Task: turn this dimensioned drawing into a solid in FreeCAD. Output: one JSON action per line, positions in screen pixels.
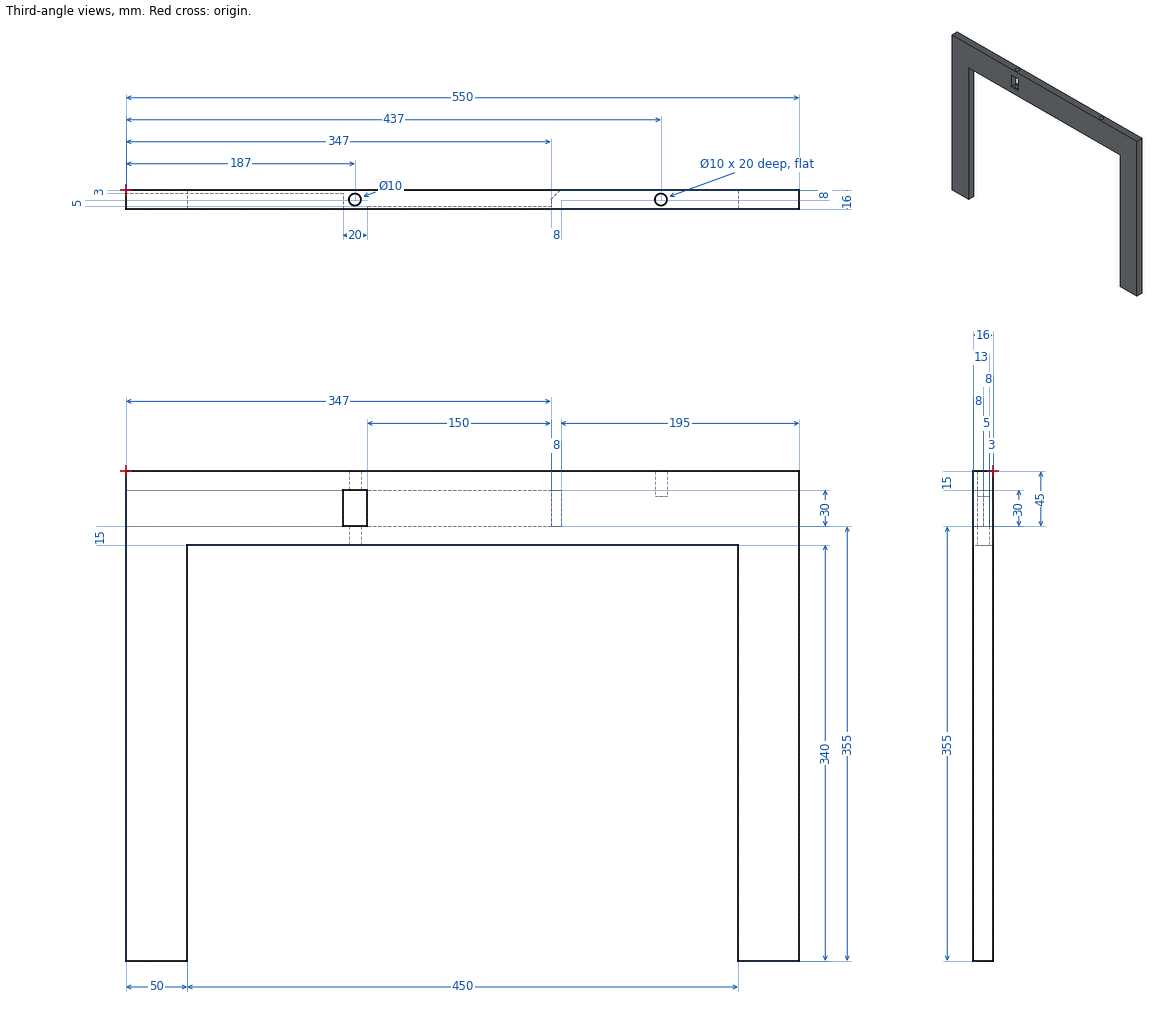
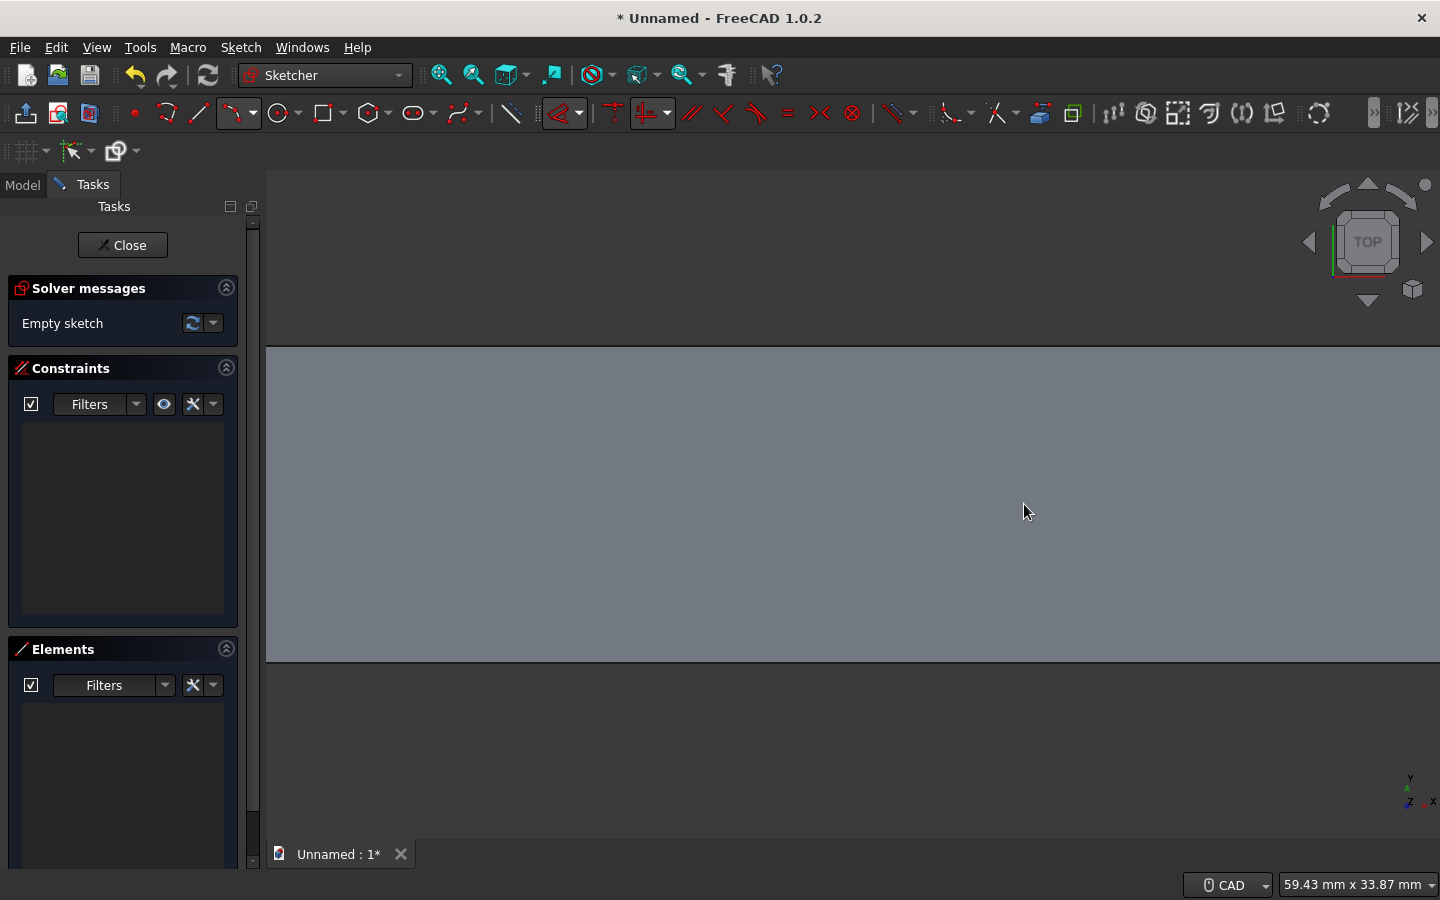
{"action": "scroll", "coordinate": [771, 504], "scroll_direction": "up", "scroll_amount": 4}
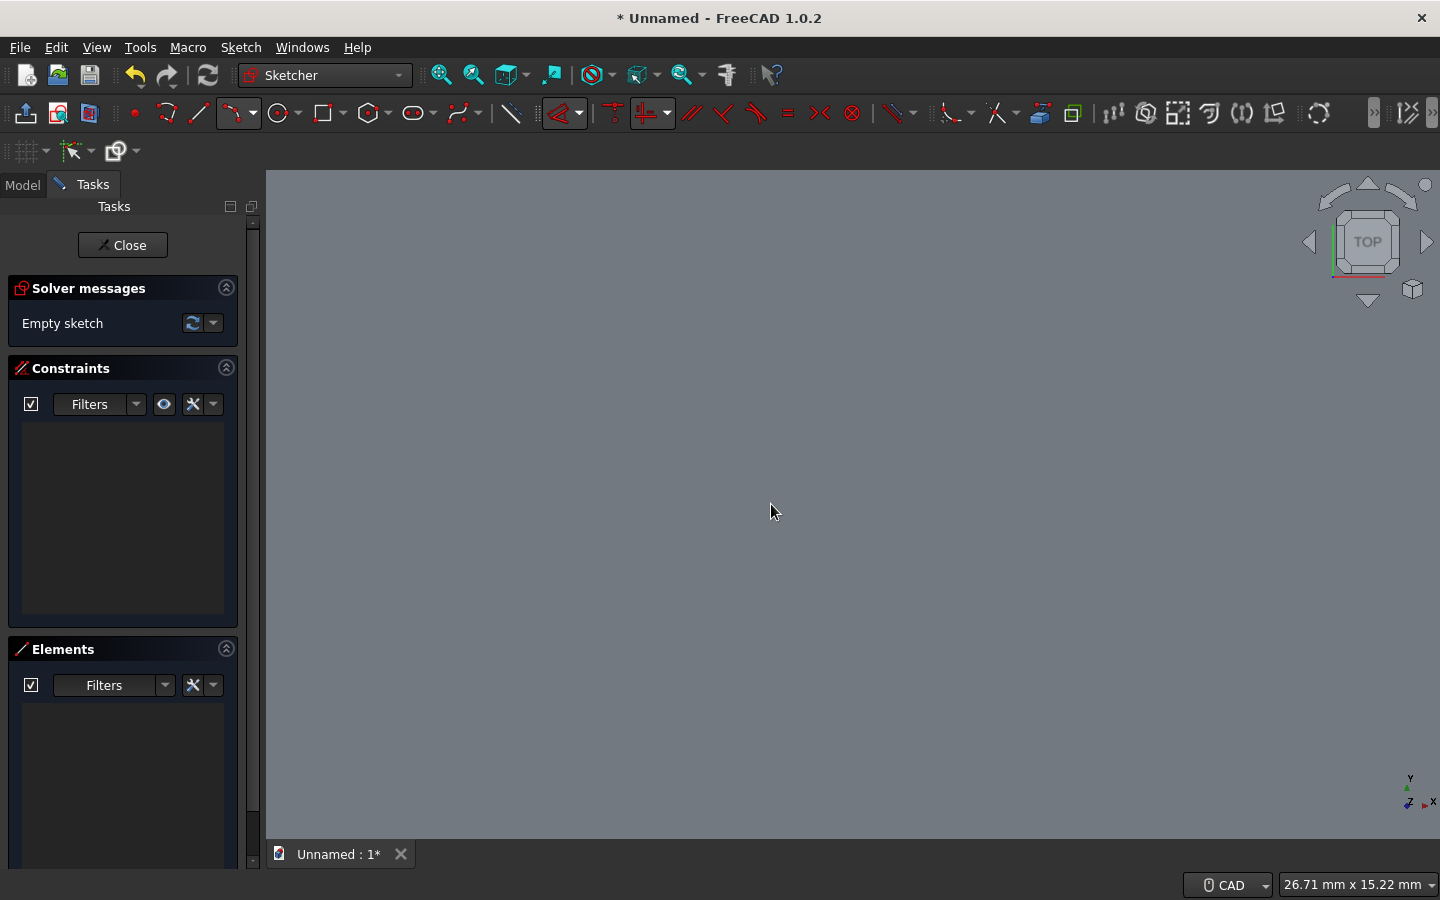
{"action": "left_click", "coordinate": [278, 114]}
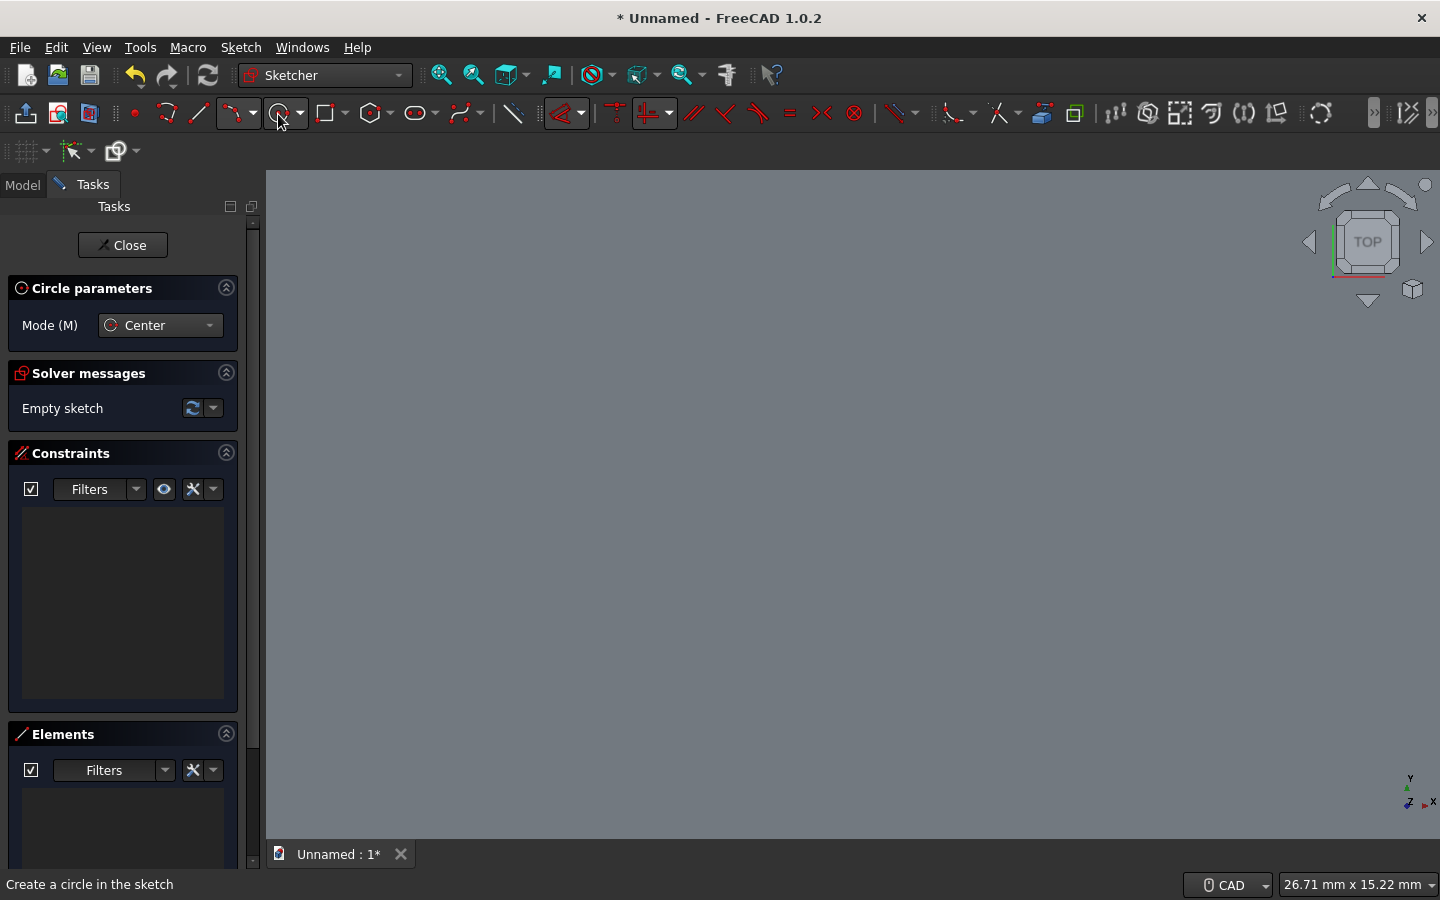
{"action": "left_click", "coordinate": [784, 504]}
{"action": "left_click", "coordinate": [939, 349]}
{"action": "key", "text": "Escape"}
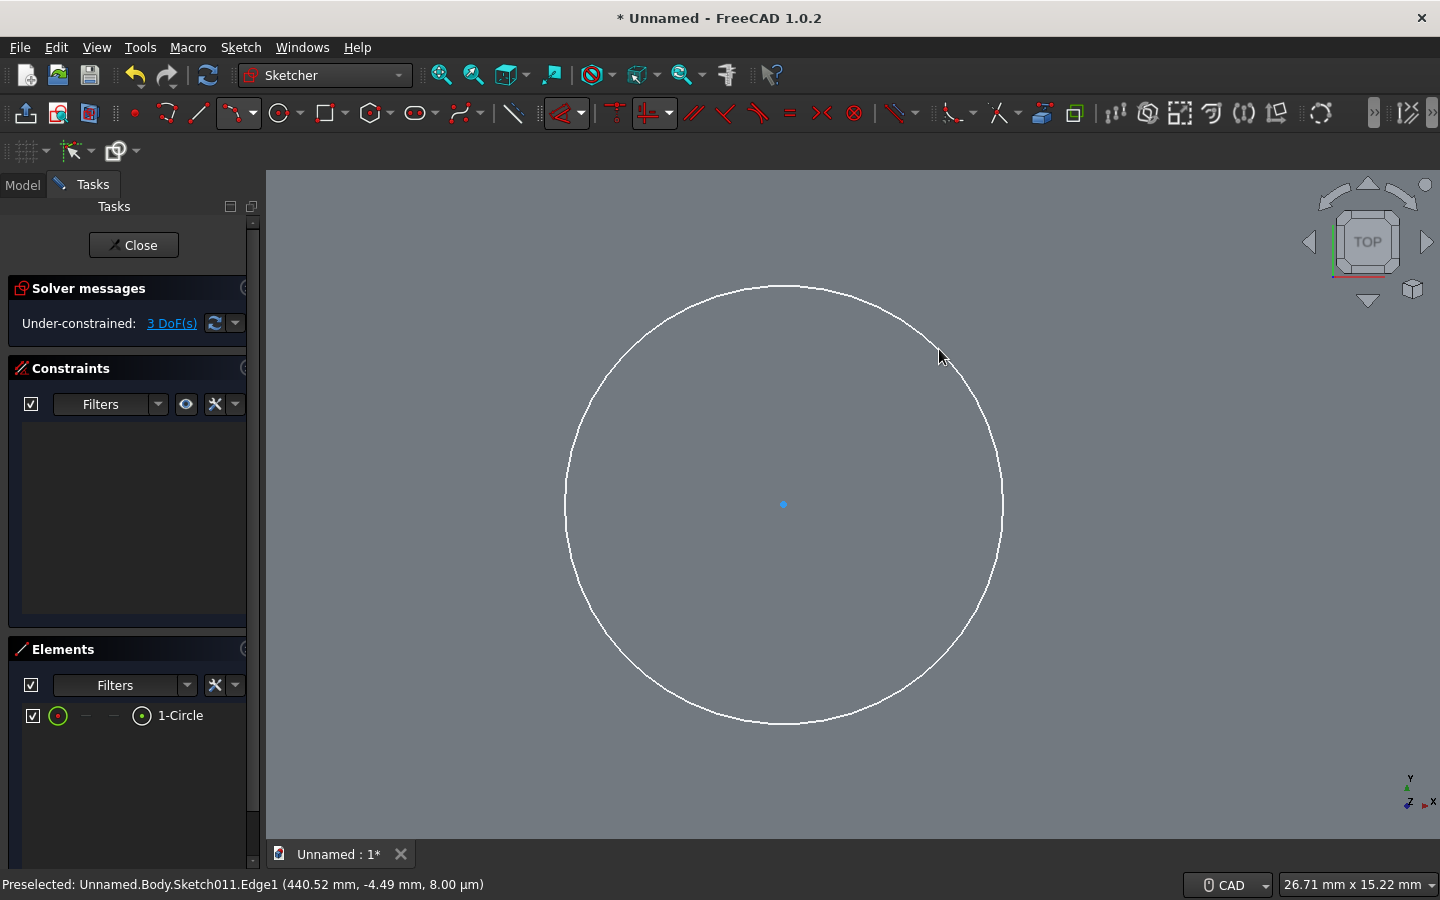
{"action": "left_click", "coordinate": [939, 350]}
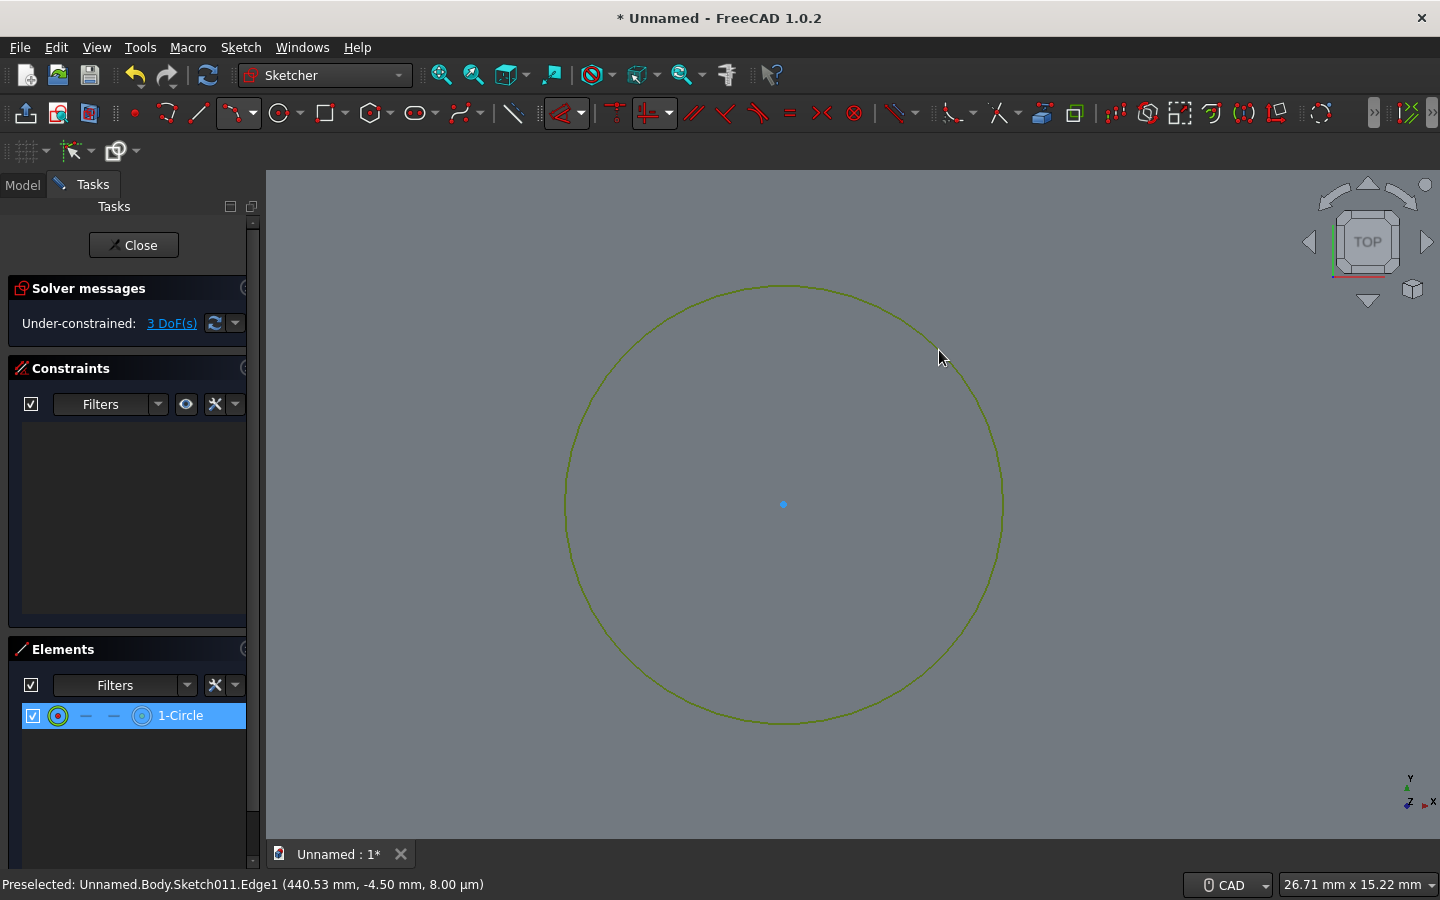
{"action": "left_click", "coordinate": [584, 114]}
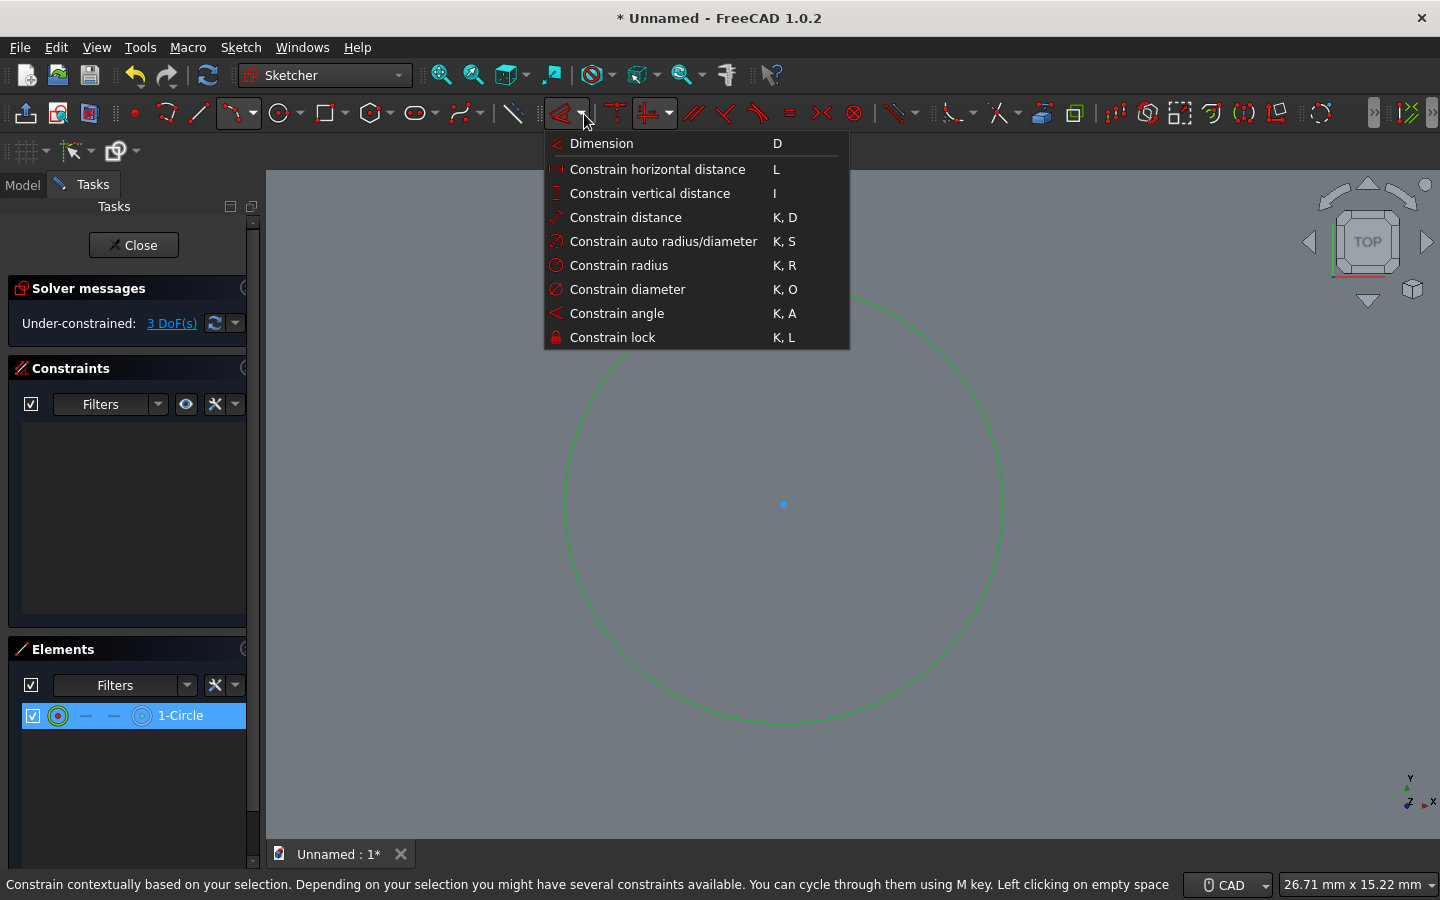
{"action": "left_click", "coordinate": [697, 289]}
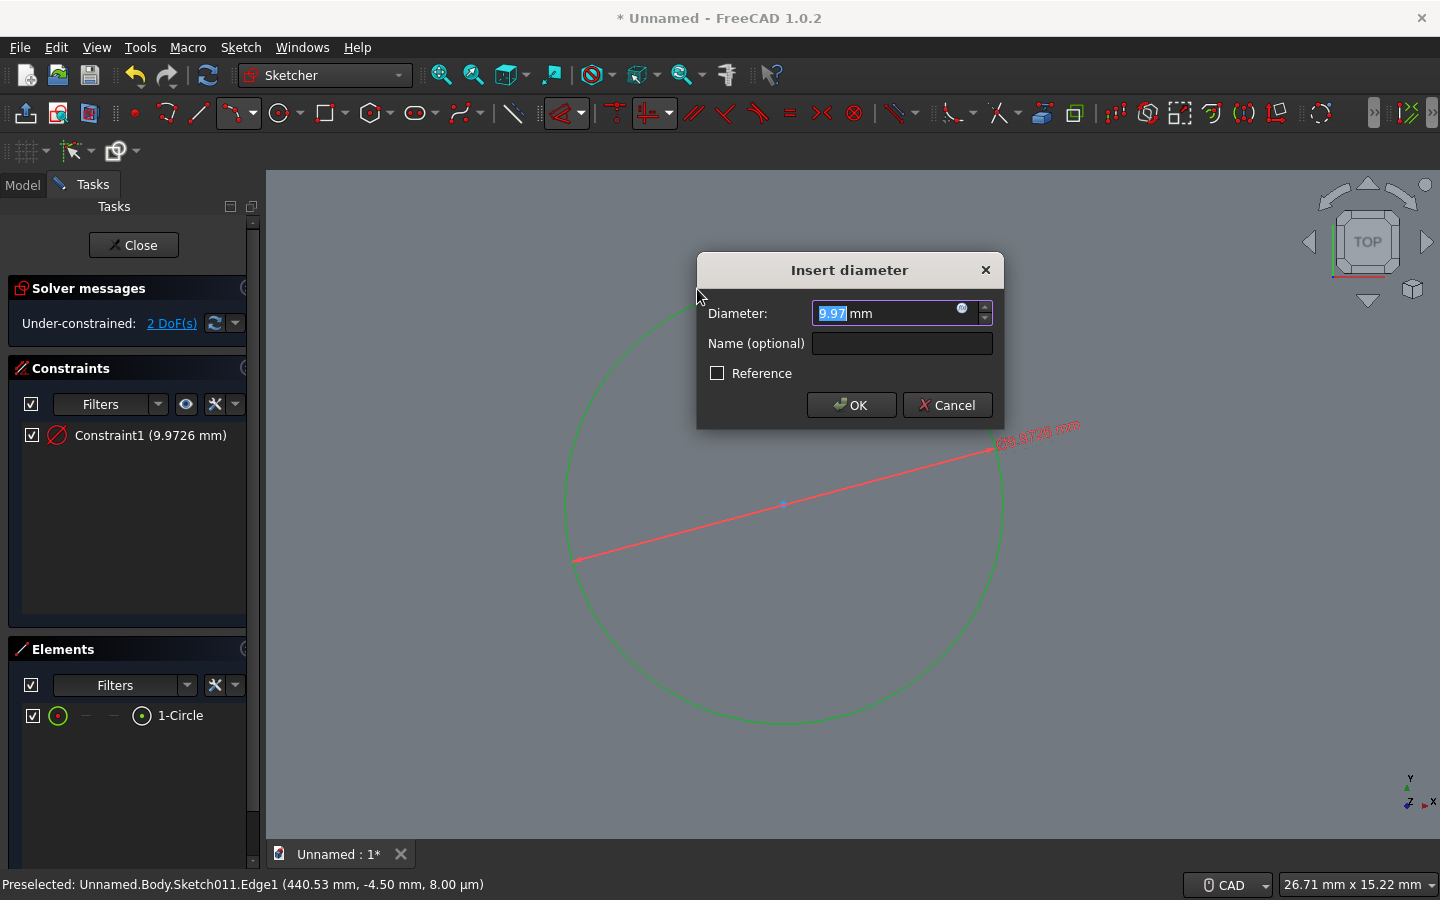
{"action": "type", "text": "10"}
{"action": "key", "text": "Return"}